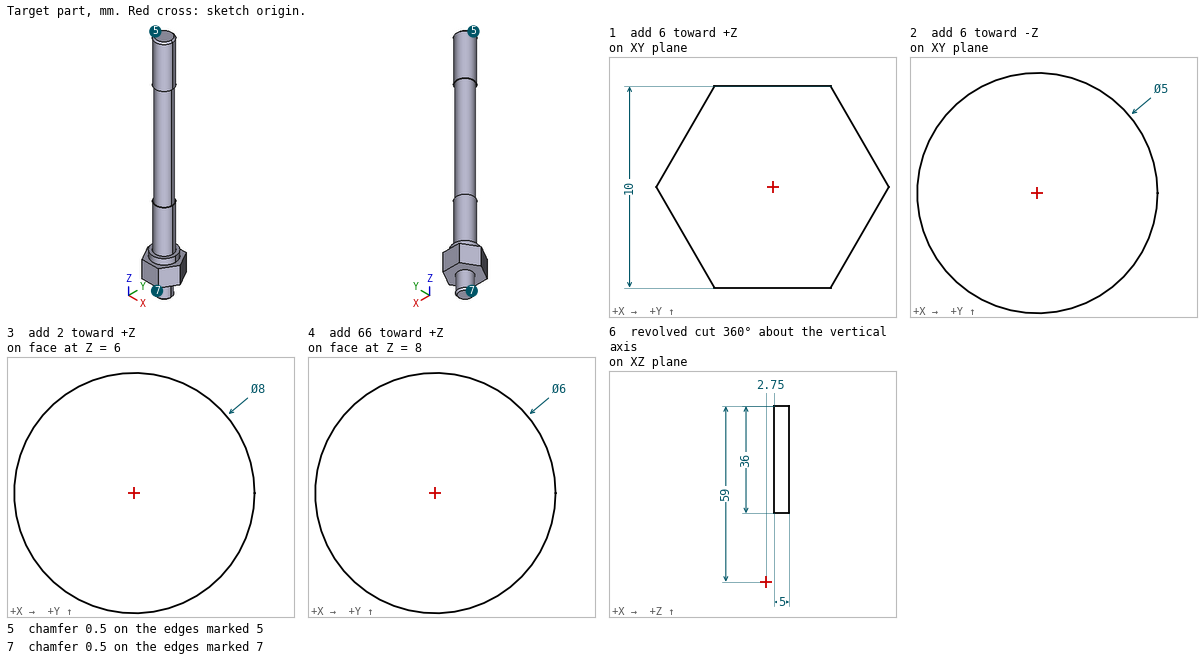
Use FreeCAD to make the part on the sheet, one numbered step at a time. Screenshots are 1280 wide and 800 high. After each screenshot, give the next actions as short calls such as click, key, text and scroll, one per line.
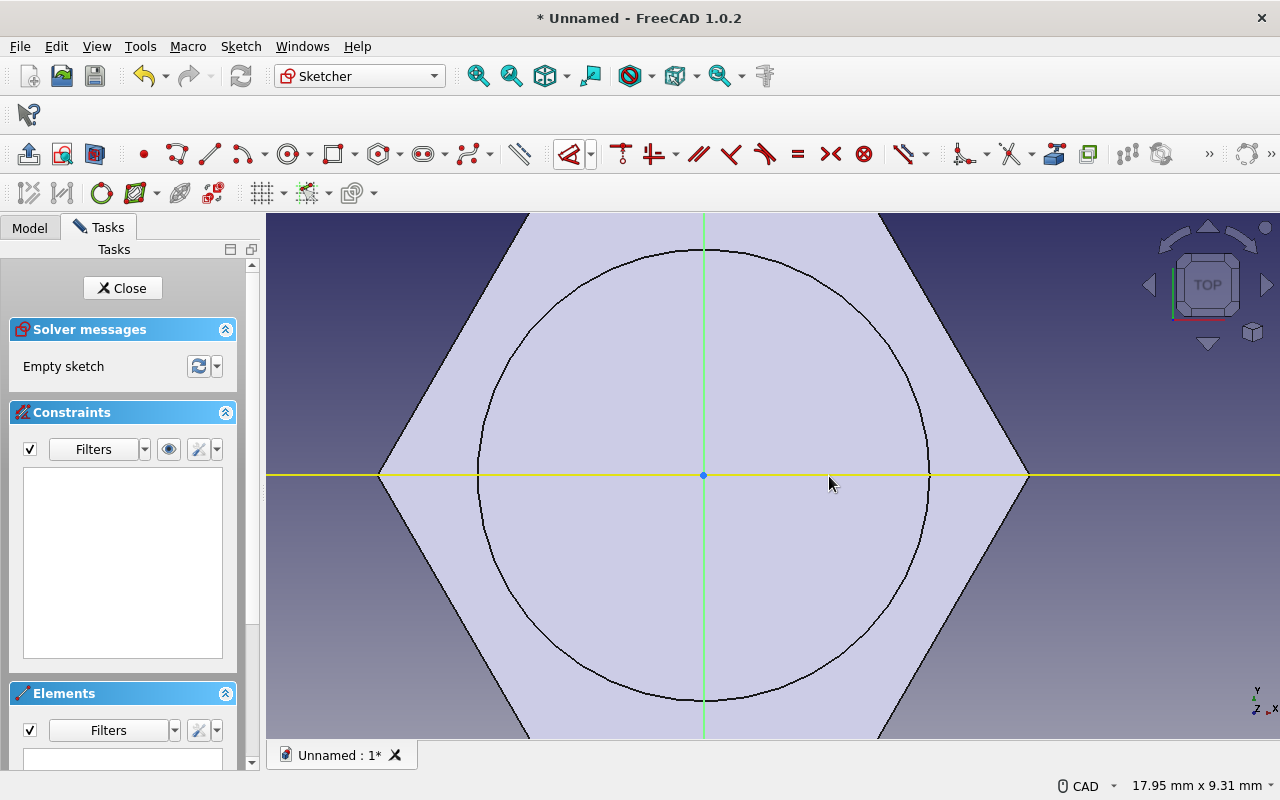
click(288, 154)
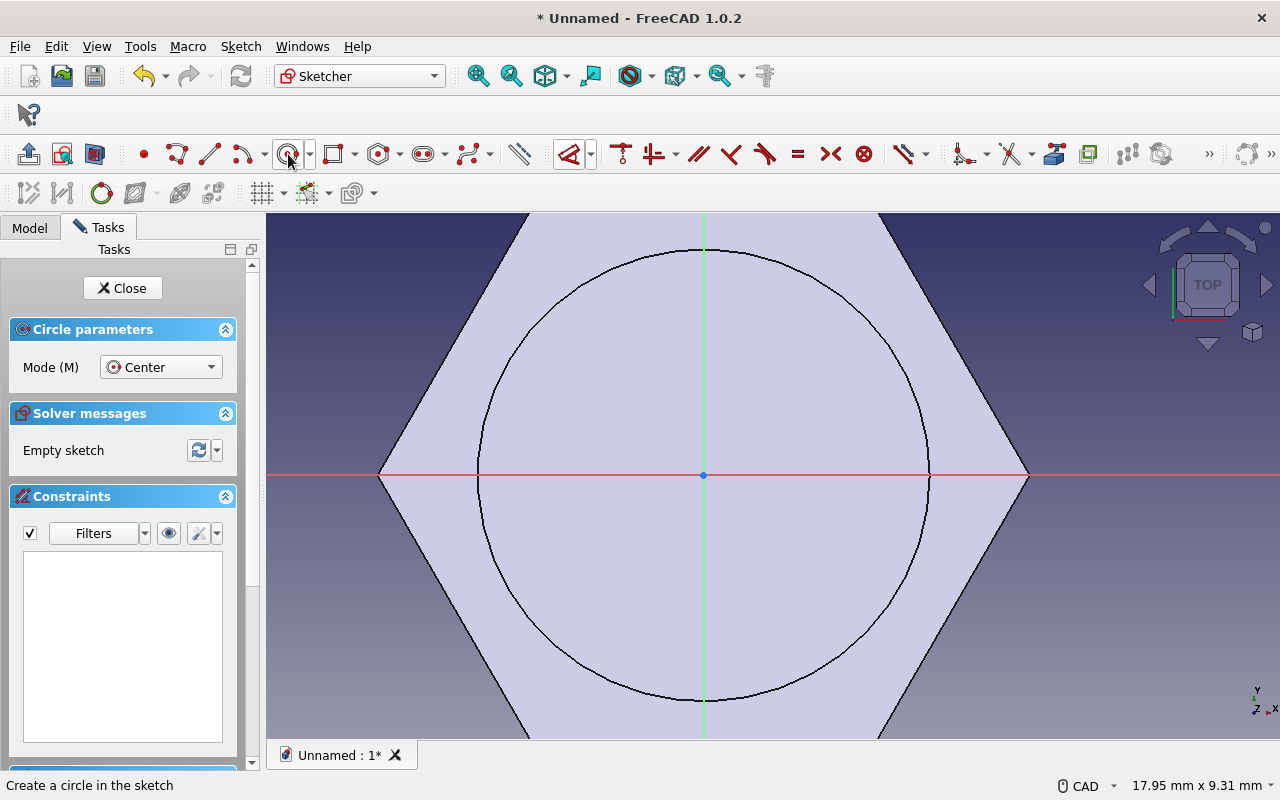
click(704, 475)
click(824, 356)
key(Escape)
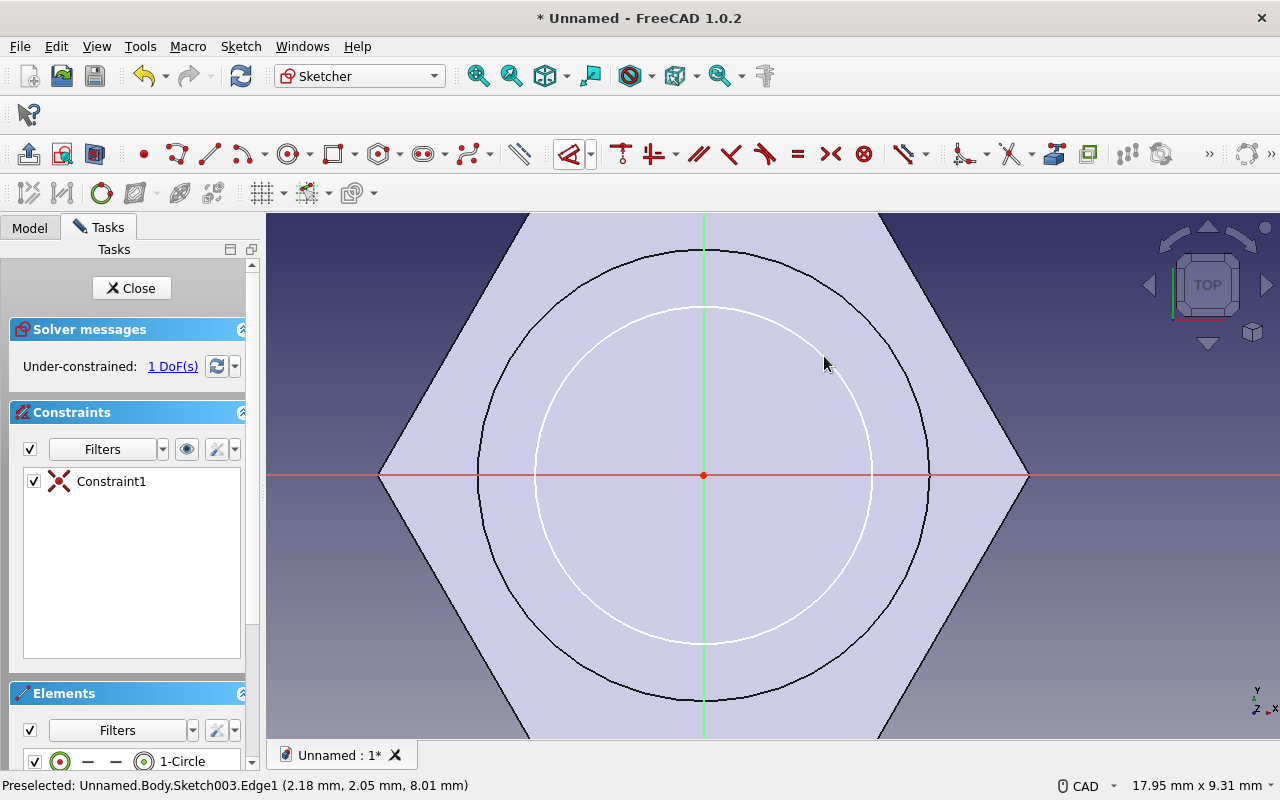
click(823, 356)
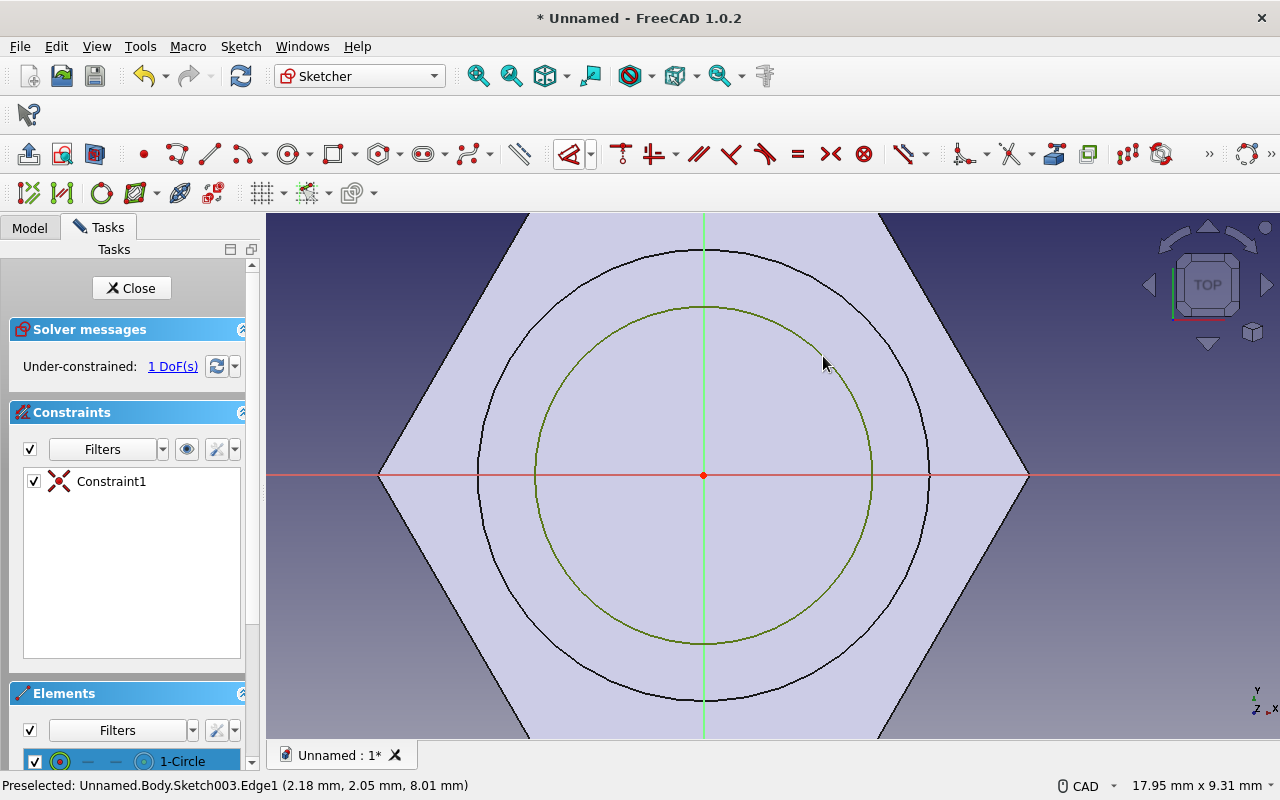
click(590, 154)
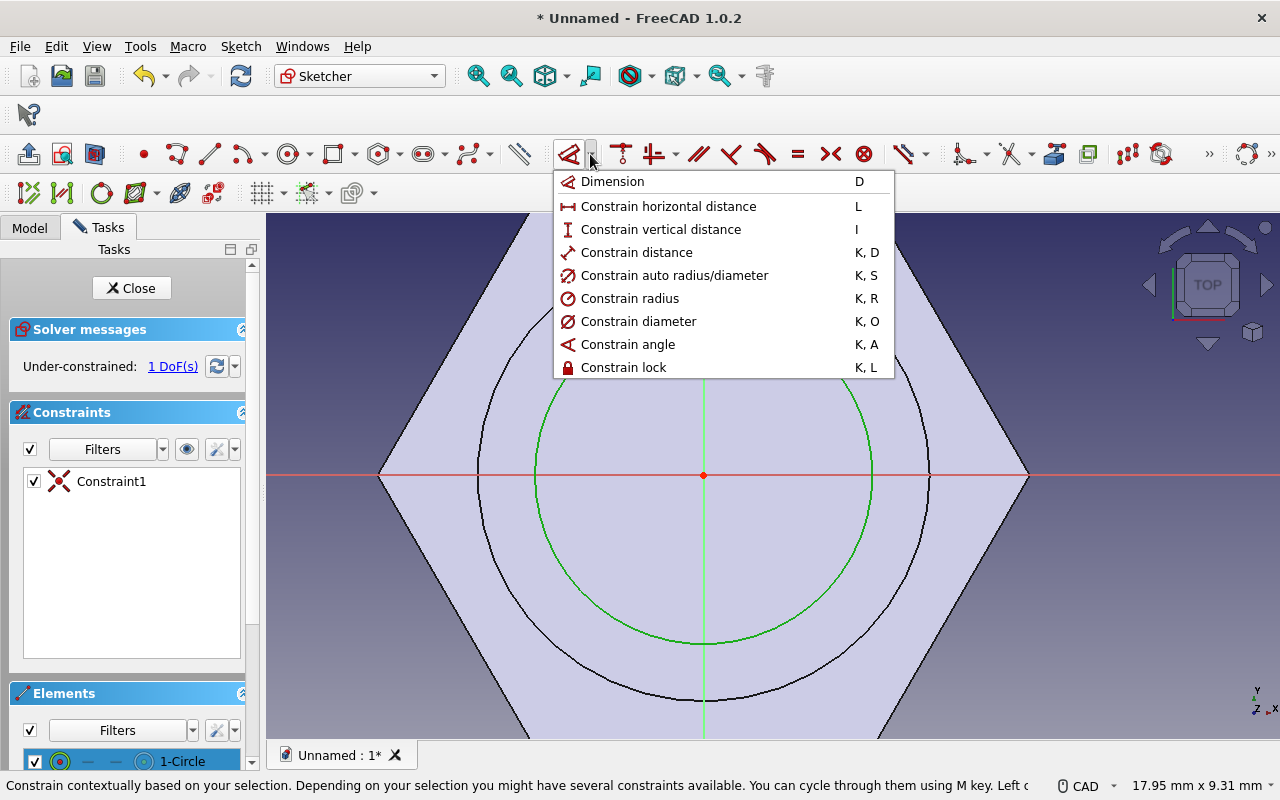
click(724, 322)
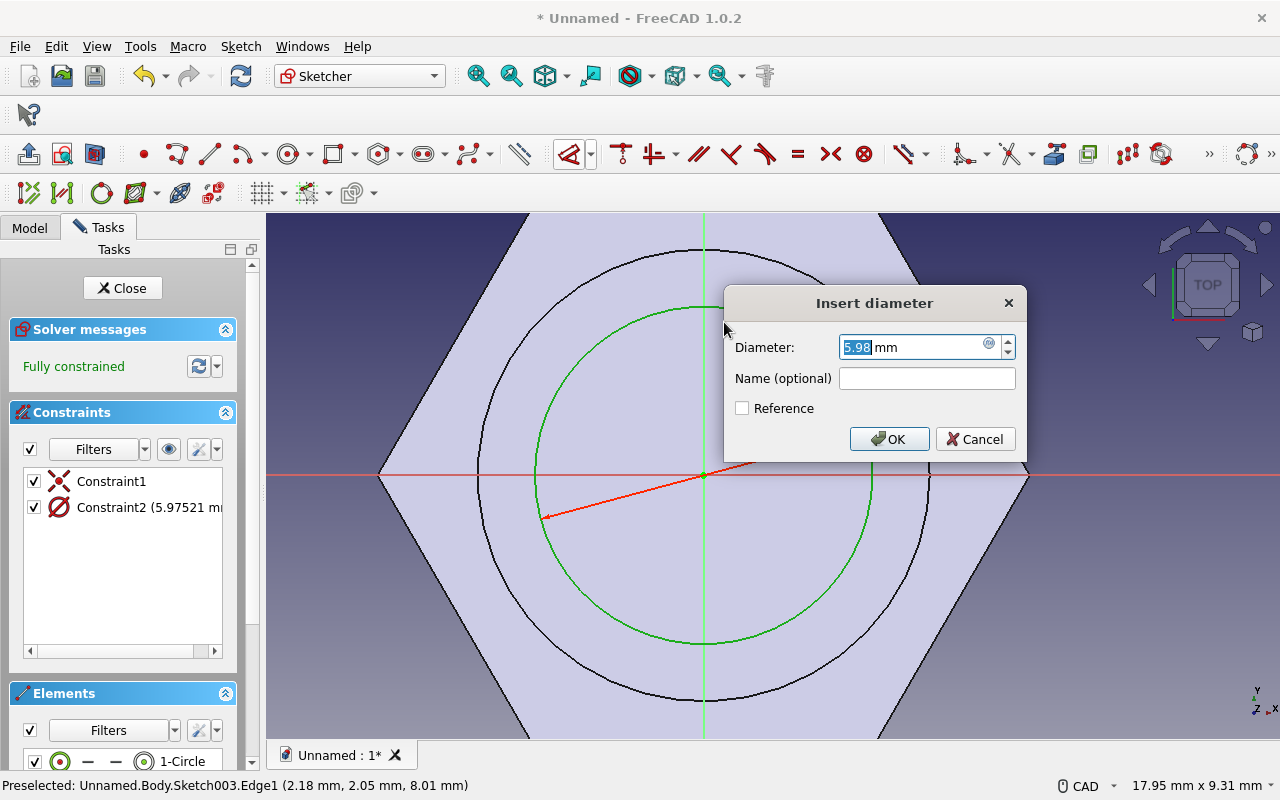
text(6)
key(Return)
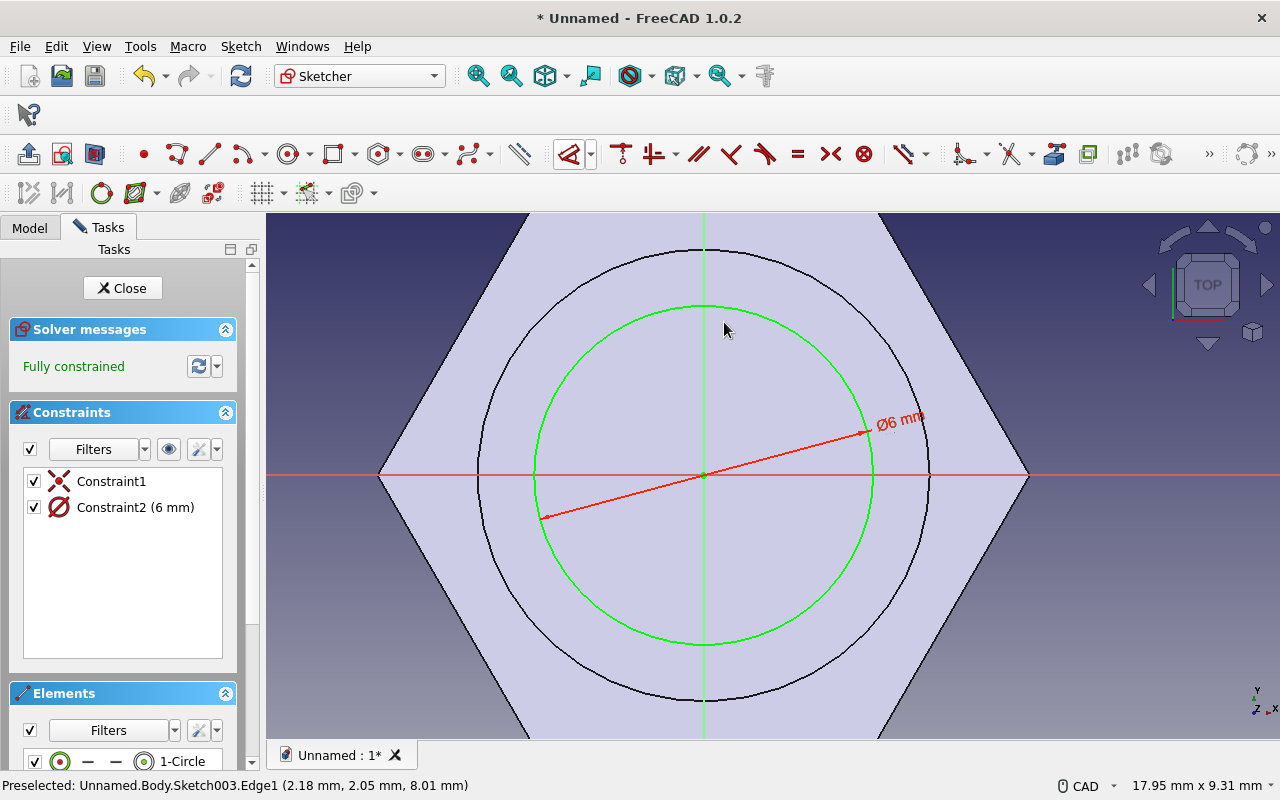
click(123, 288)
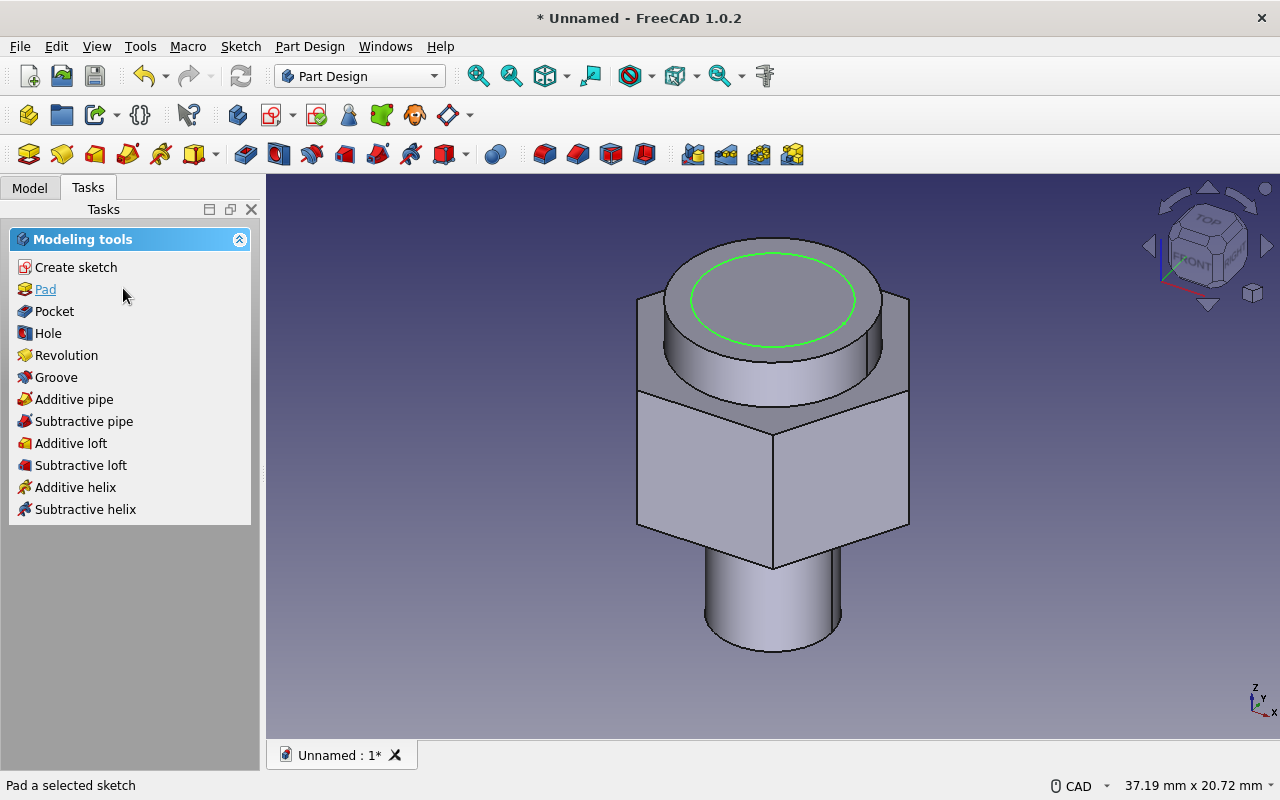
click(29, 154)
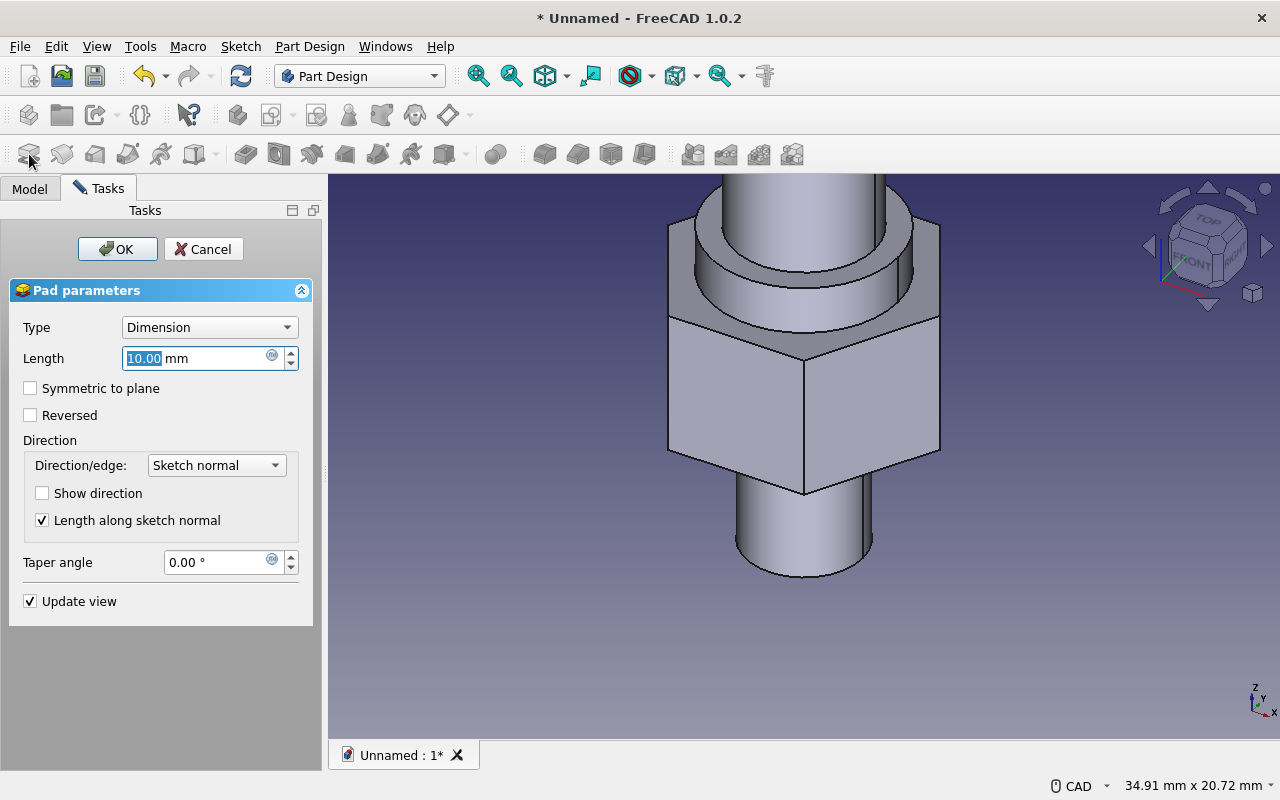
text(66)
key(Tab)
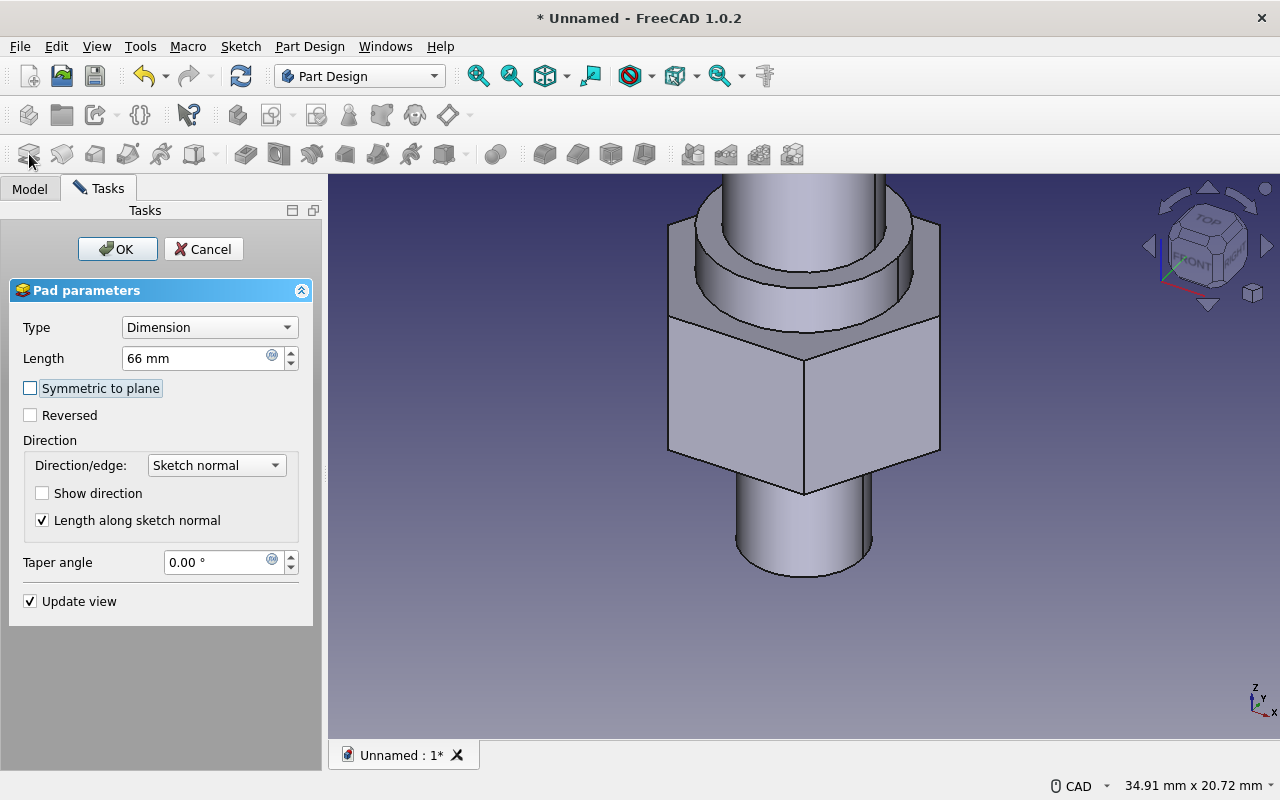
click(118, 249)